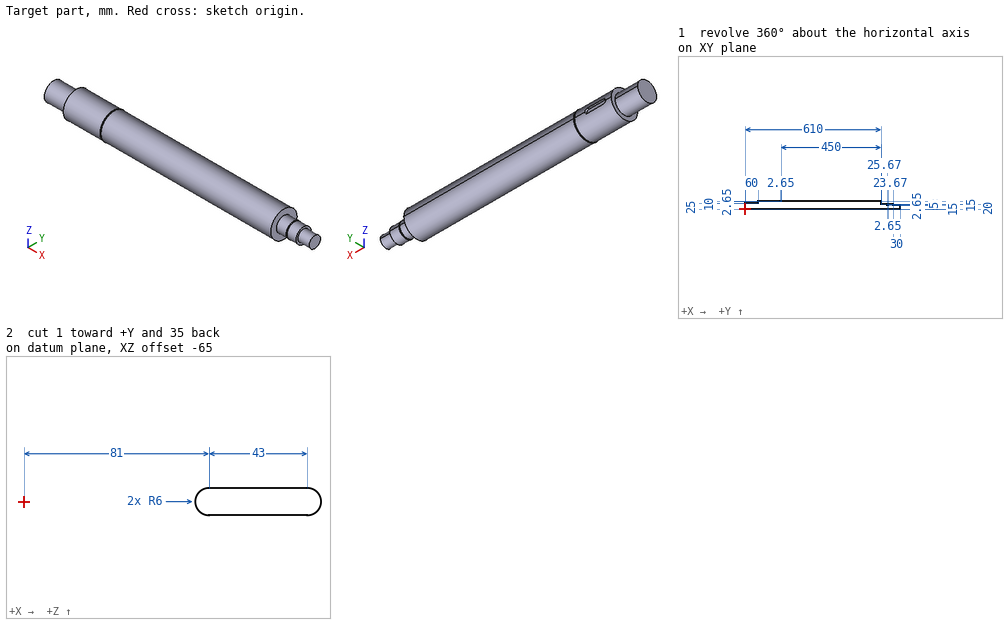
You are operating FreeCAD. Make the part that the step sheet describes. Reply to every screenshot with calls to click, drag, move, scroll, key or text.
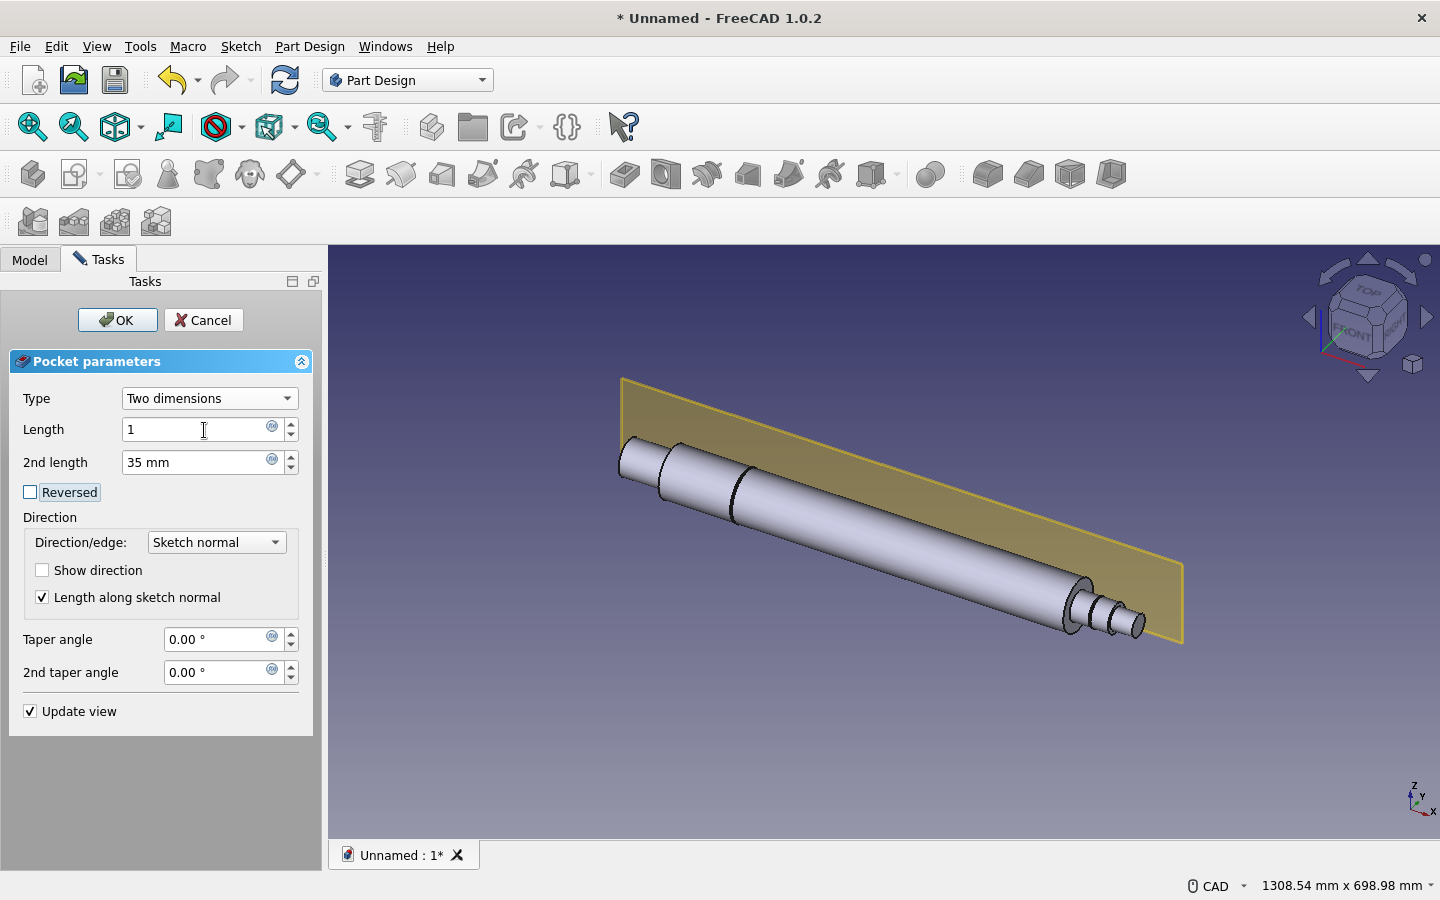
click(118, 320)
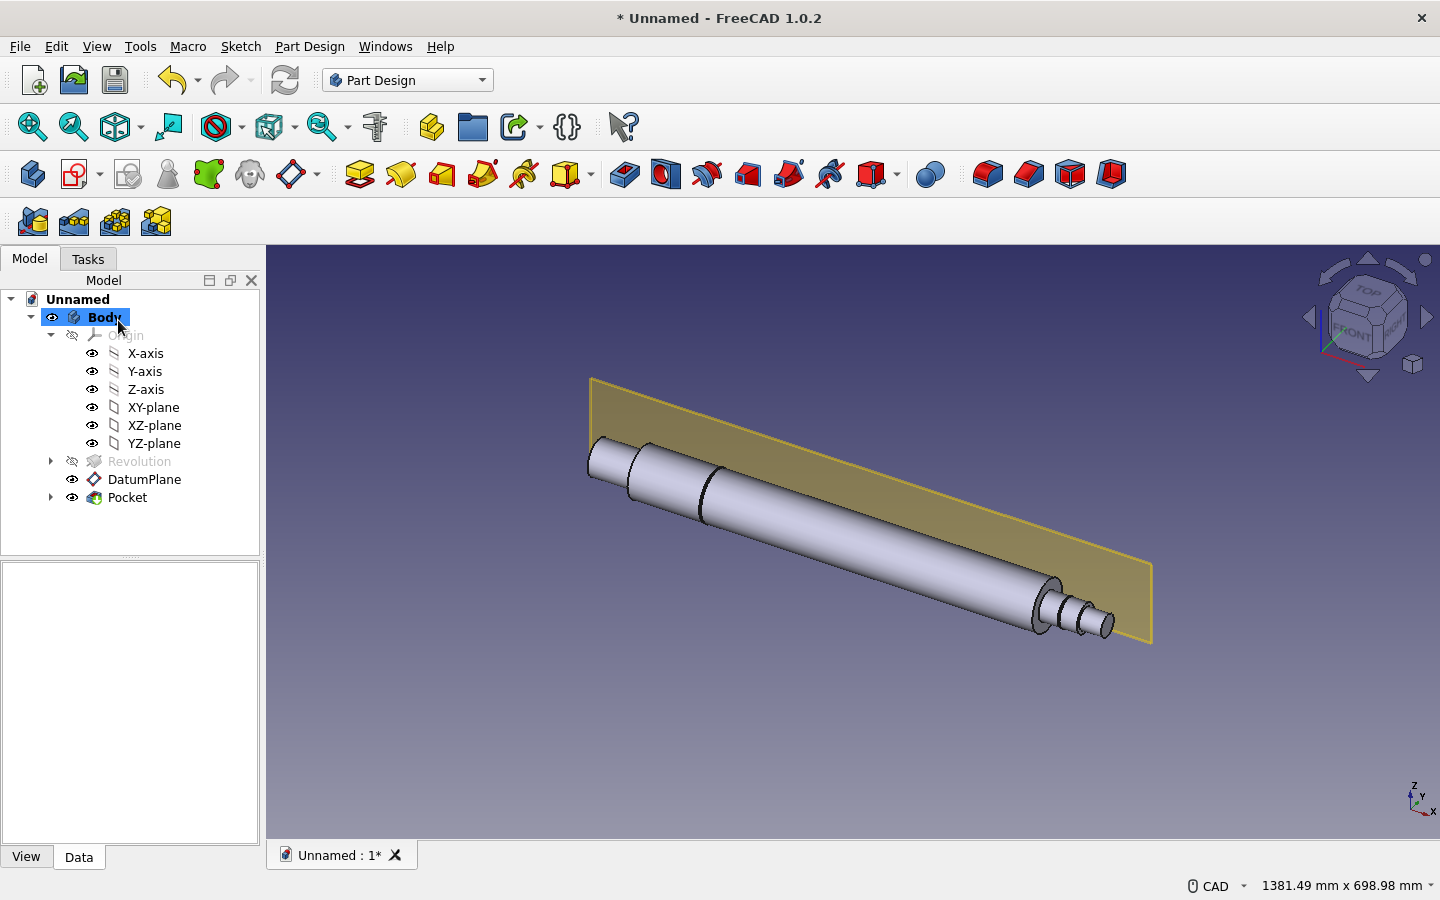
click(117, 479)
key(space)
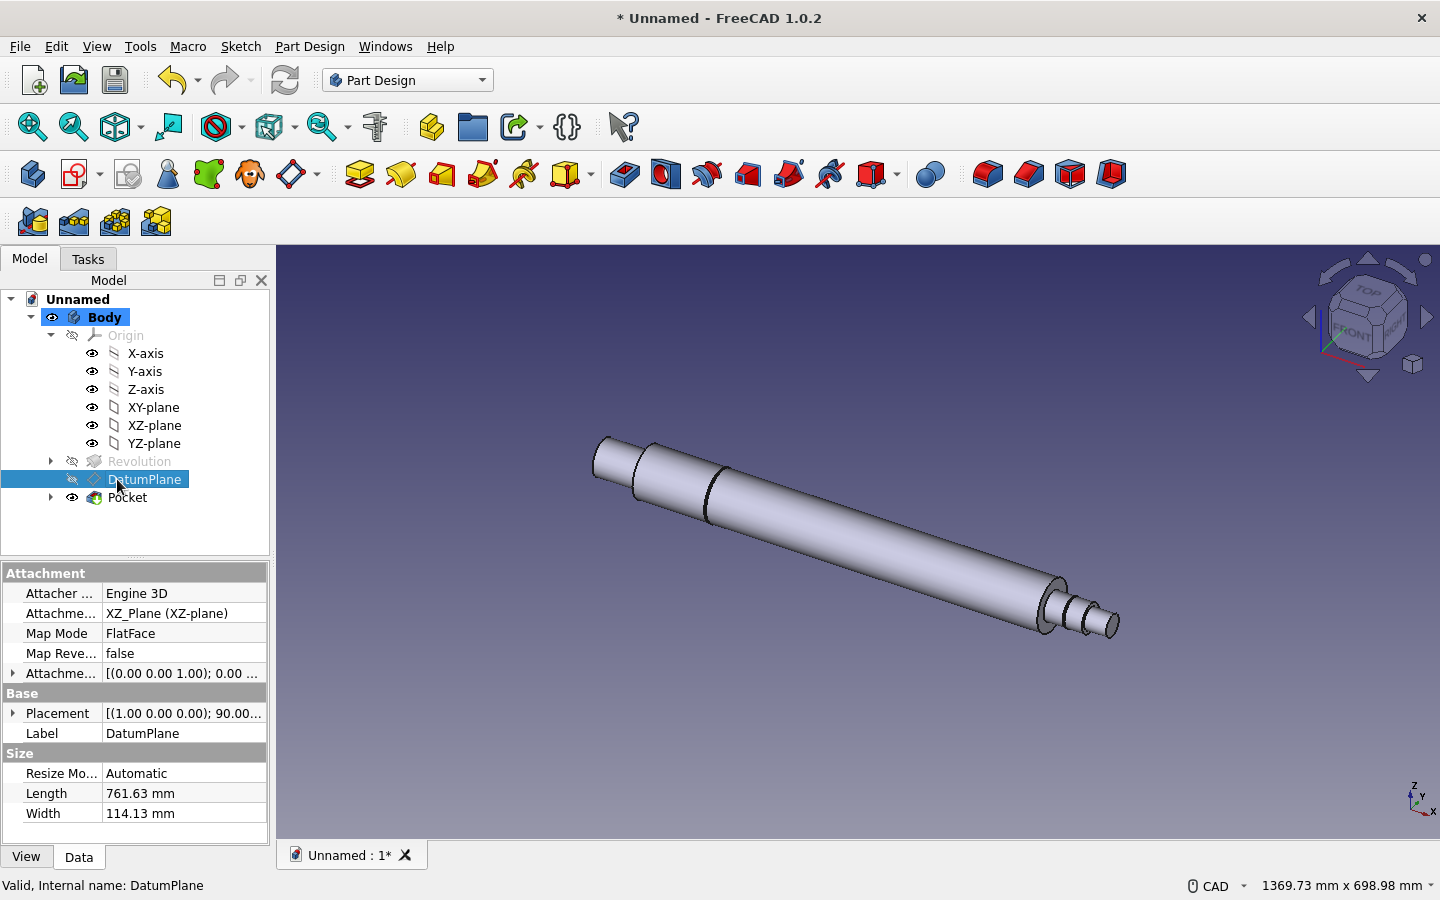
key(0)